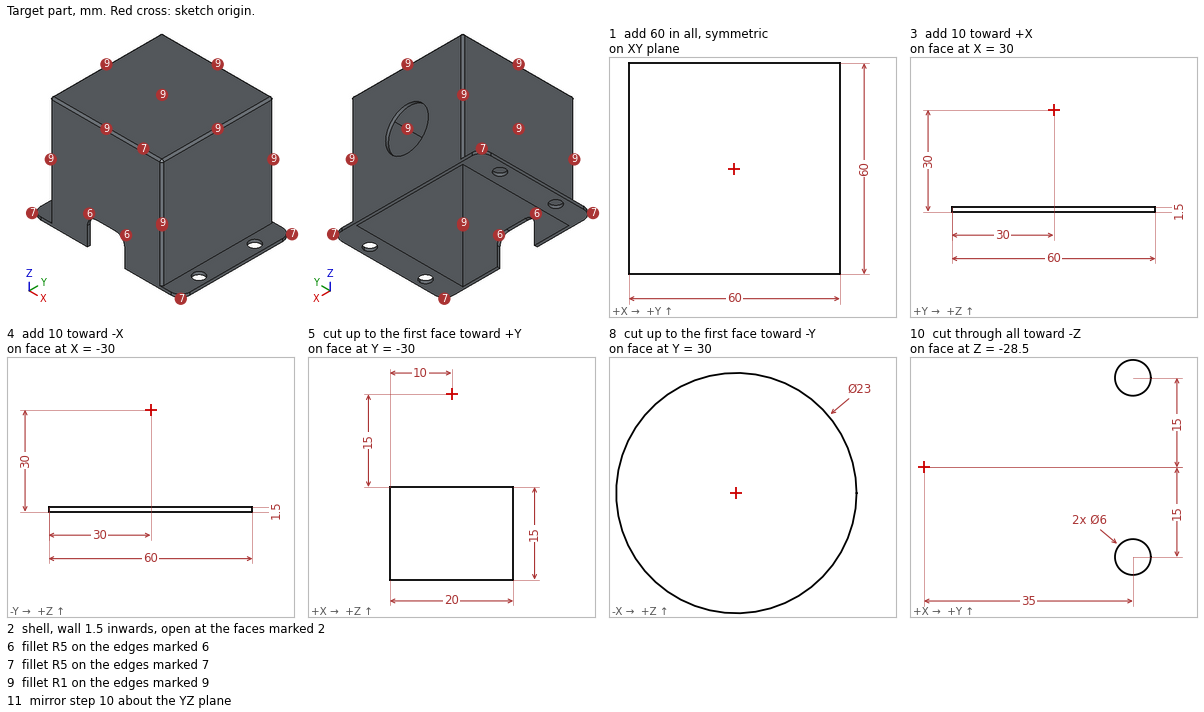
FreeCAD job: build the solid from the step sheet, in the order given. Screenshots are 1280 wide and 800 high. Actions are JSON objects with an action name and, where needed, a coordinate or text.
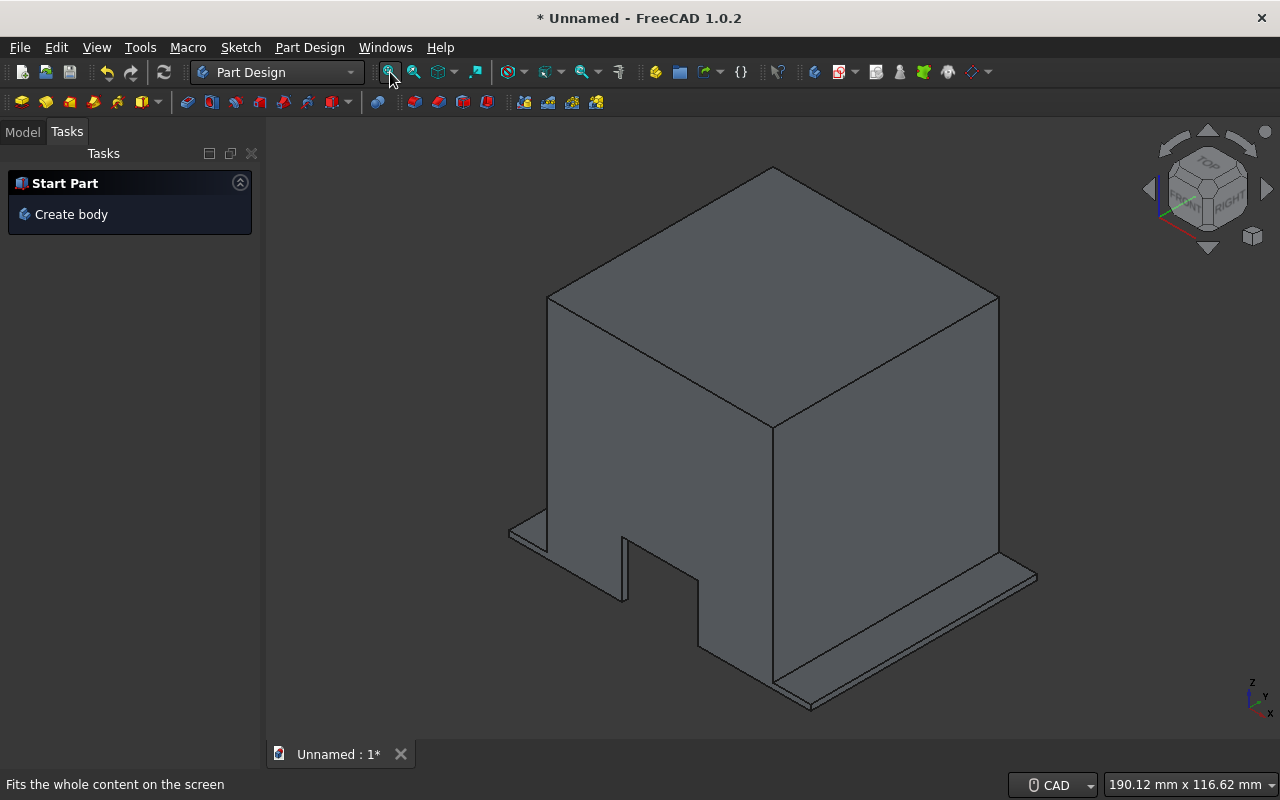
{"action": "key", "text": "2"}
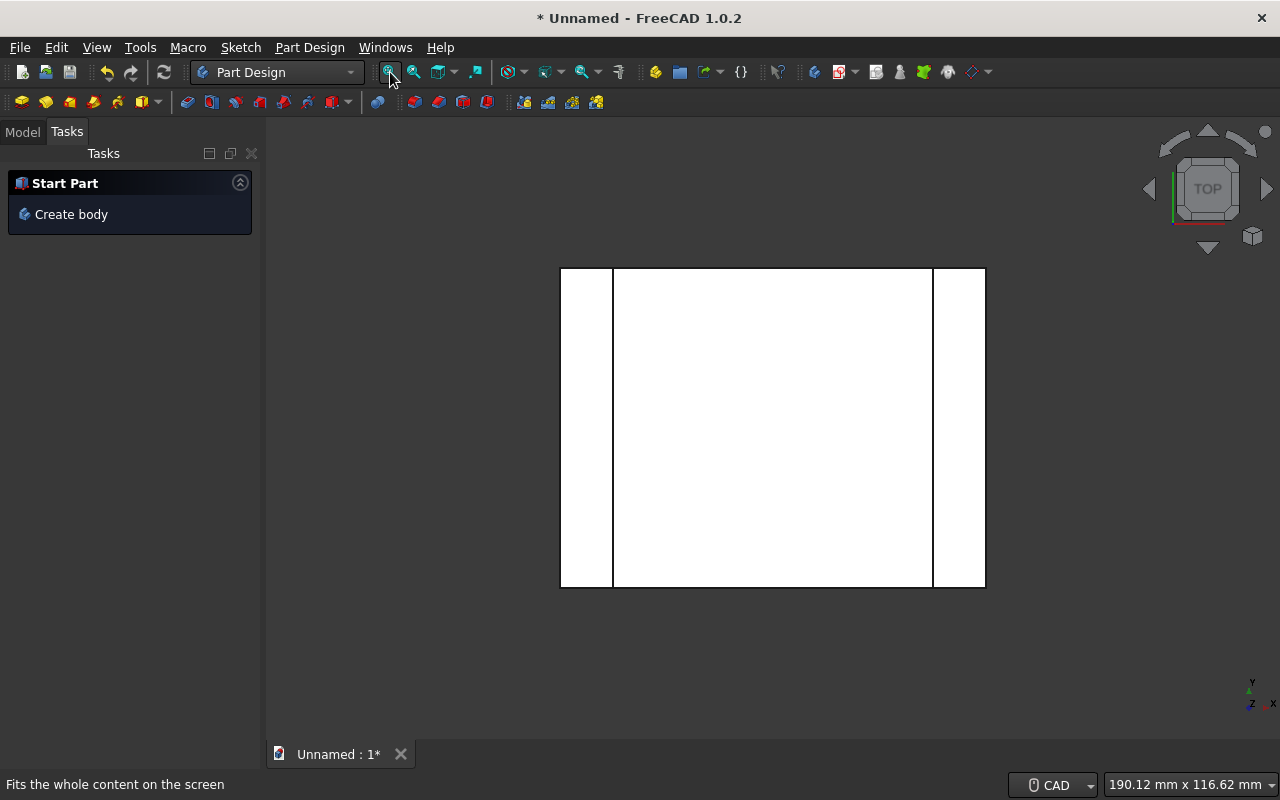
{"action": "scroll", "coordinate": [826, 583], "scroll_direction": "up", "scroll_amount": 9}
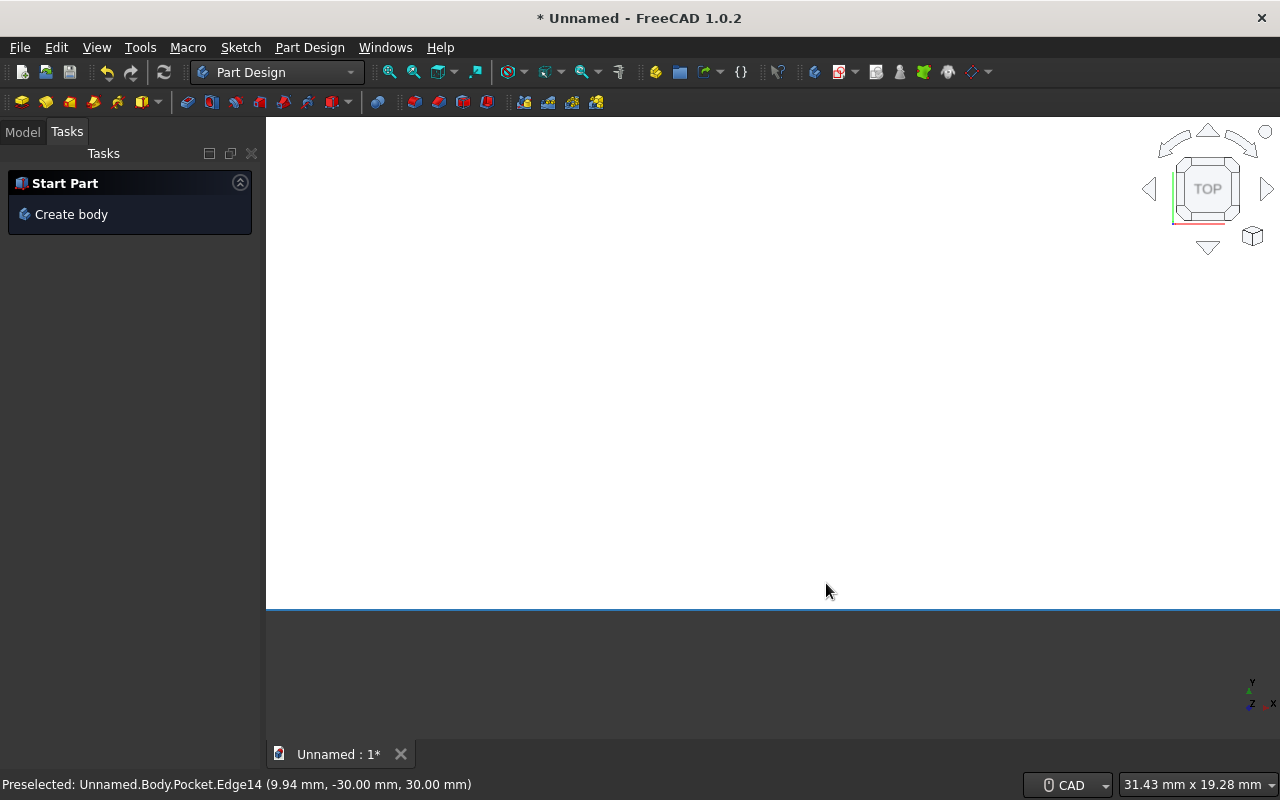
{"action": "key", "text": "v f"}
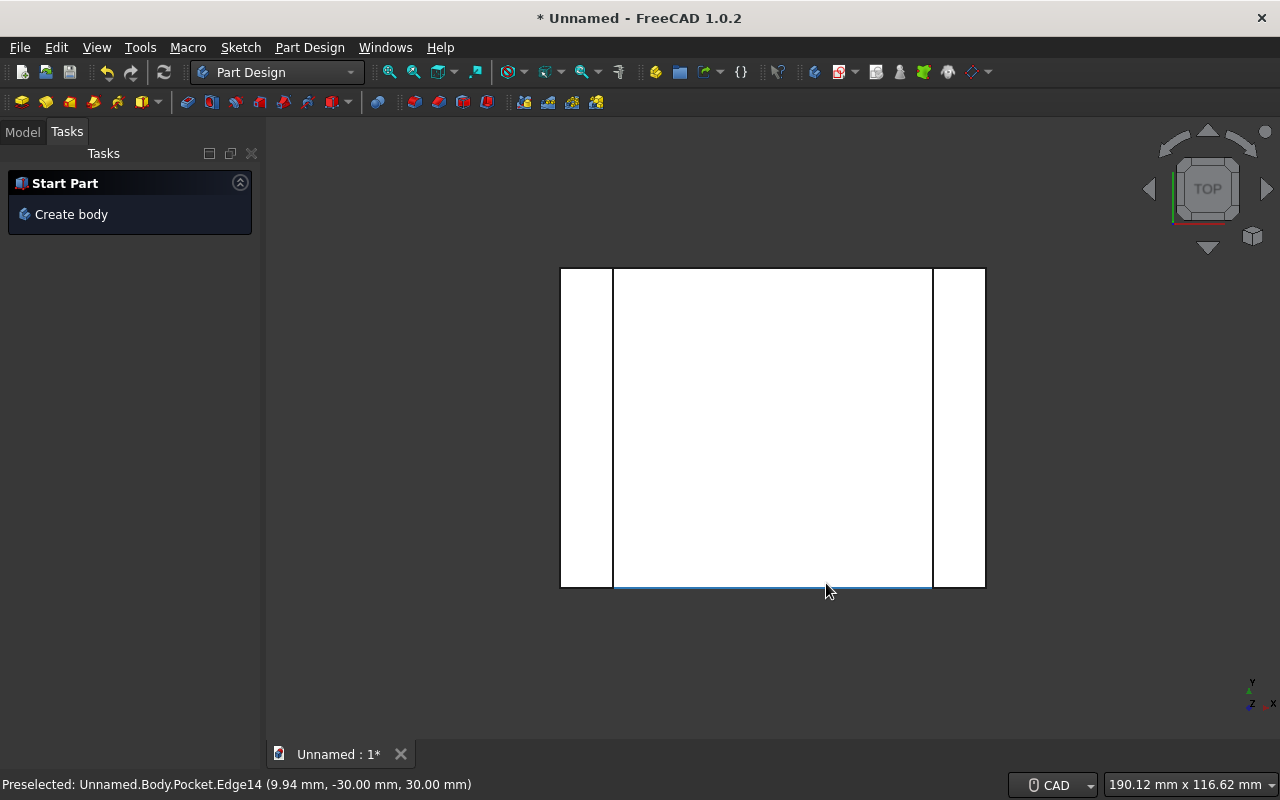
{"action": "key", "text": "0"}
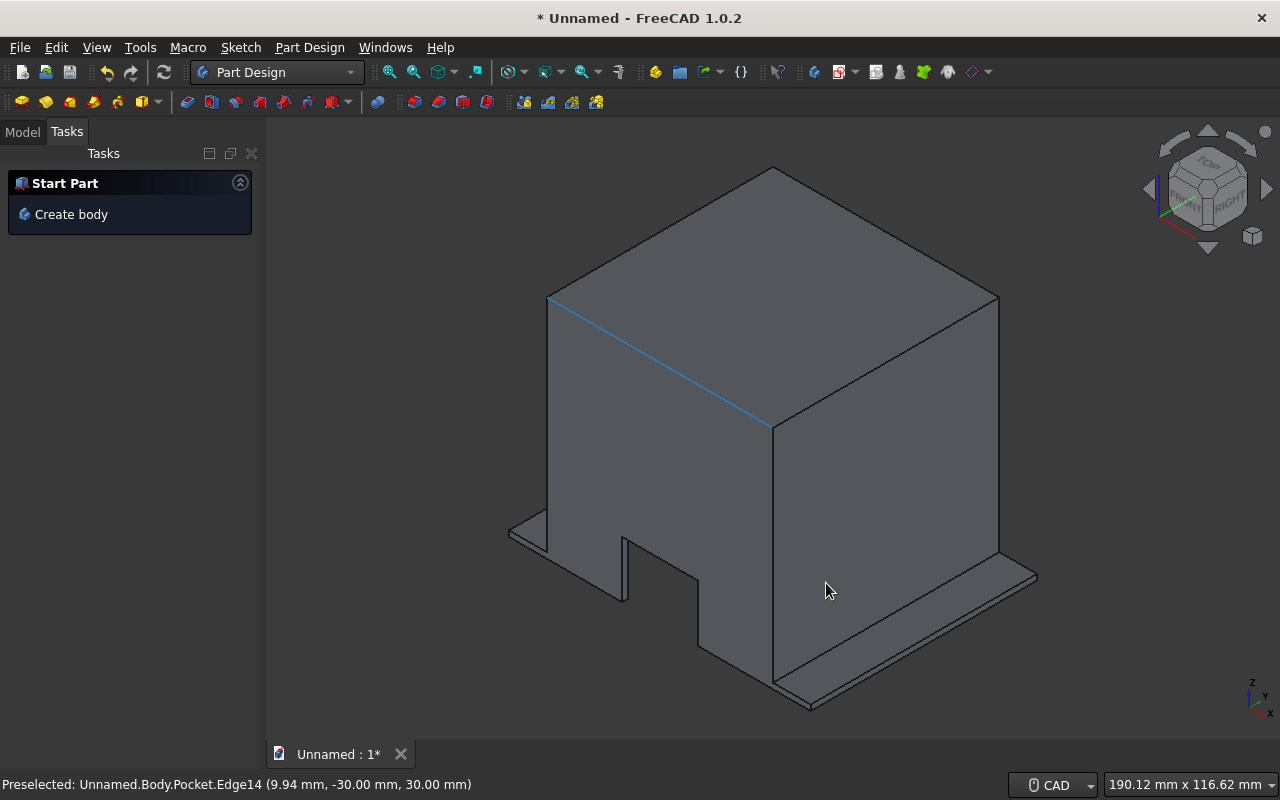
{"action": "scroll", "coordinate": [700, 578], "scroll_direction": "up", "scroll_amount": 9}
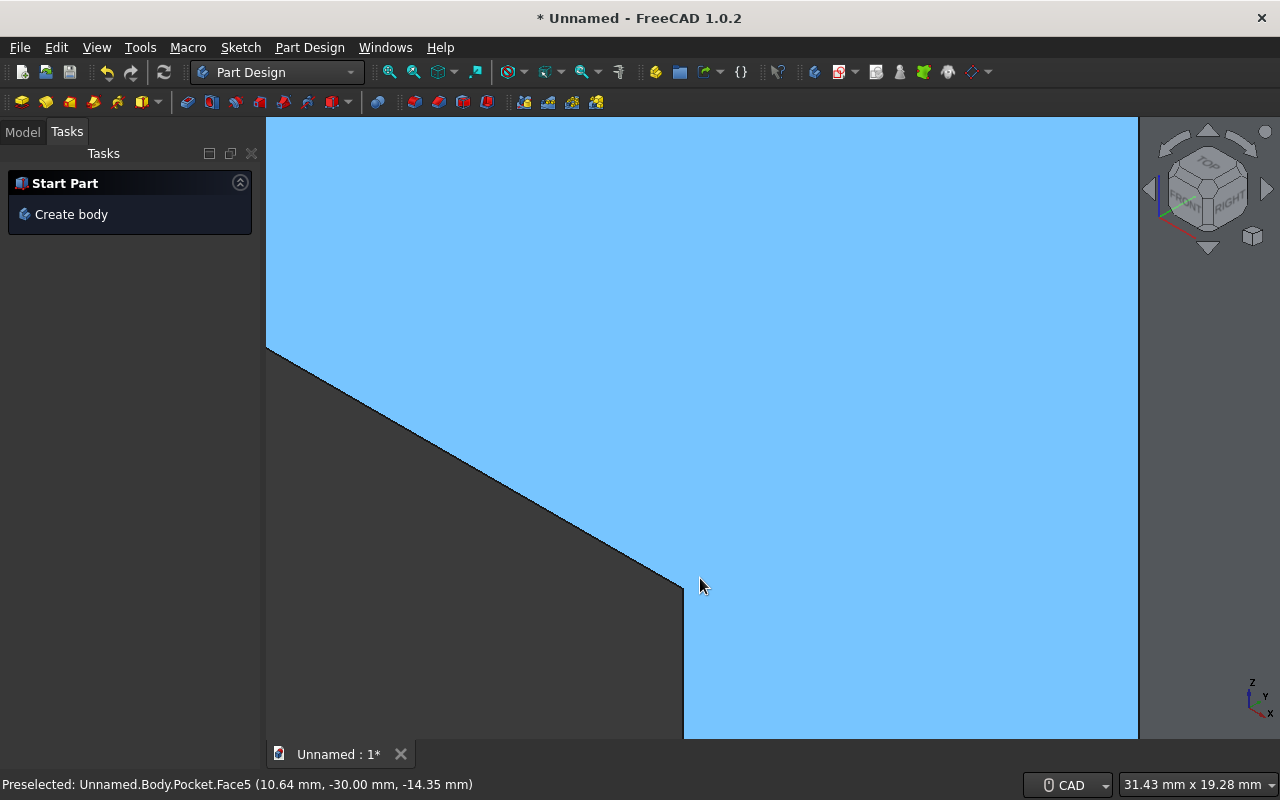
{"action": "left_click", "coordinate": [390, 72]}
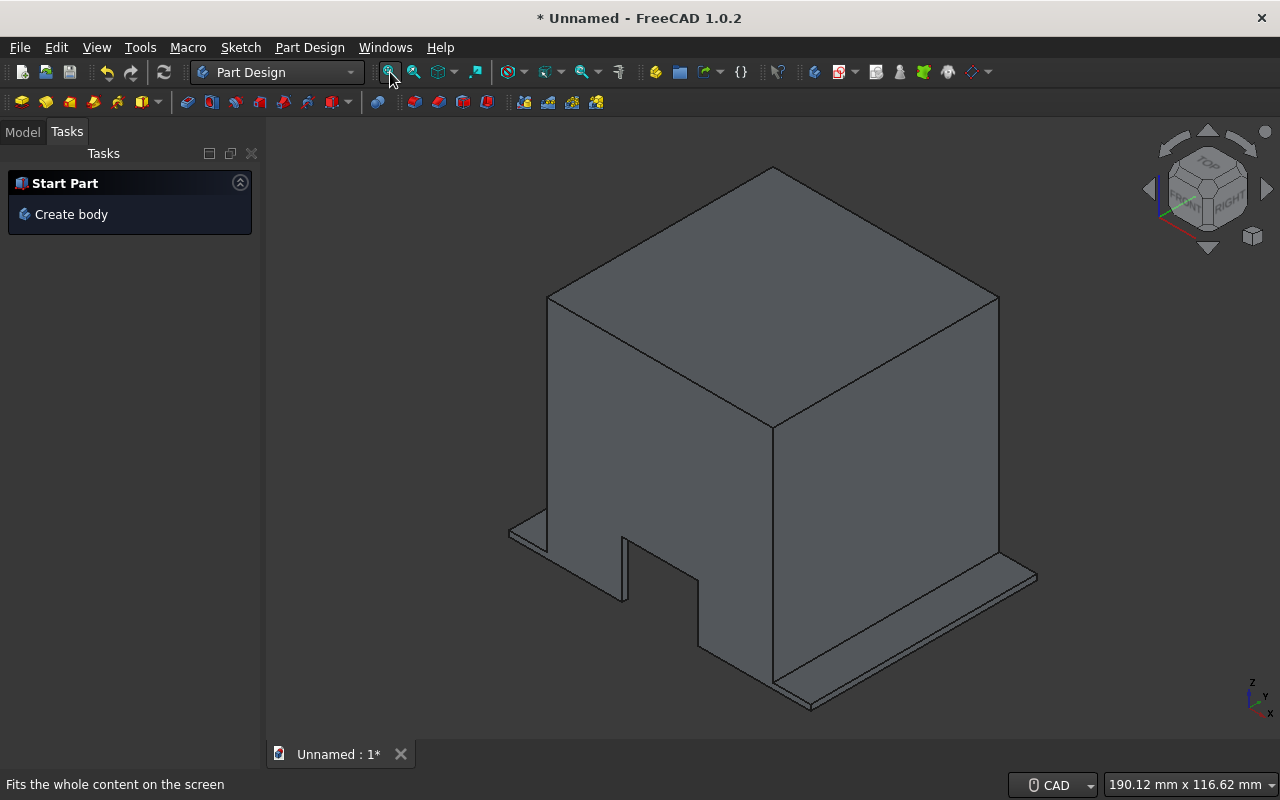
{"action": "key", "text": "1"}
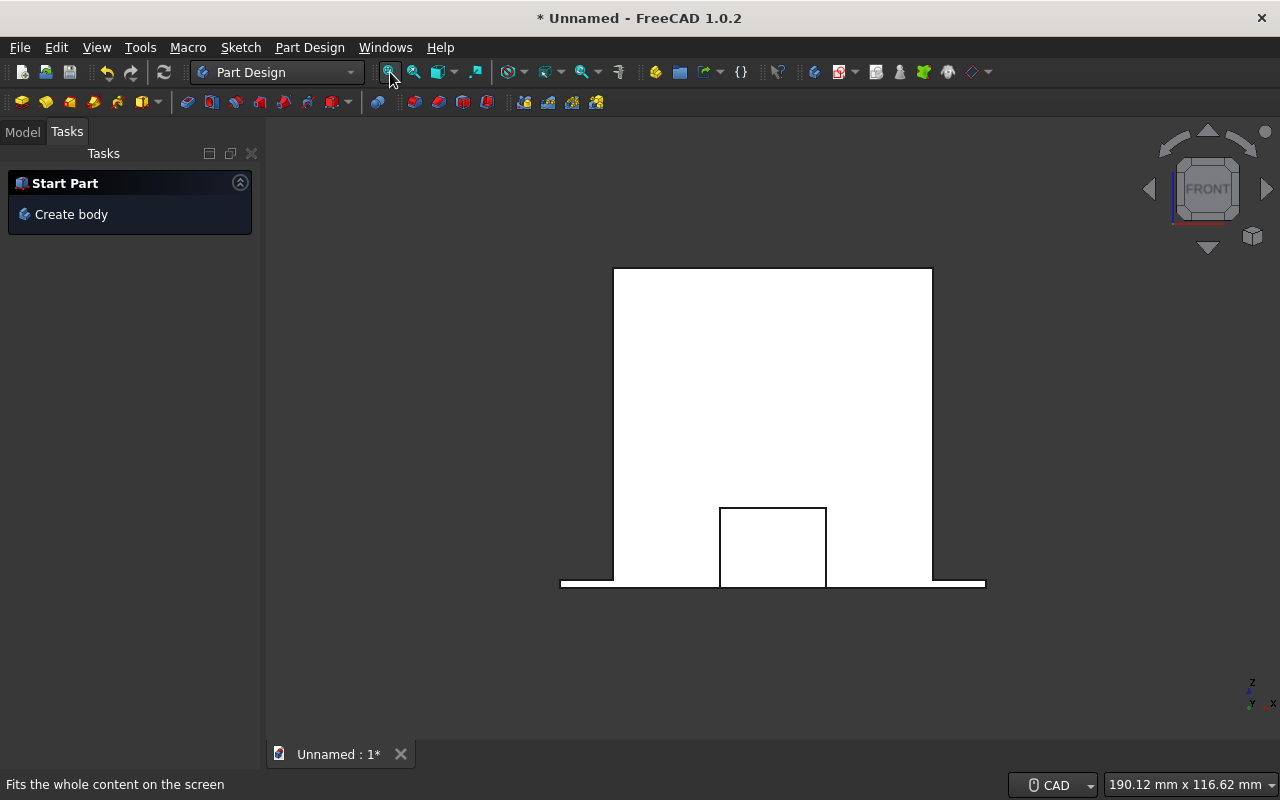
{"action": "scroll", "coordinate": [826, 507], "scroll_direction": "up", "scroll_amount": 9}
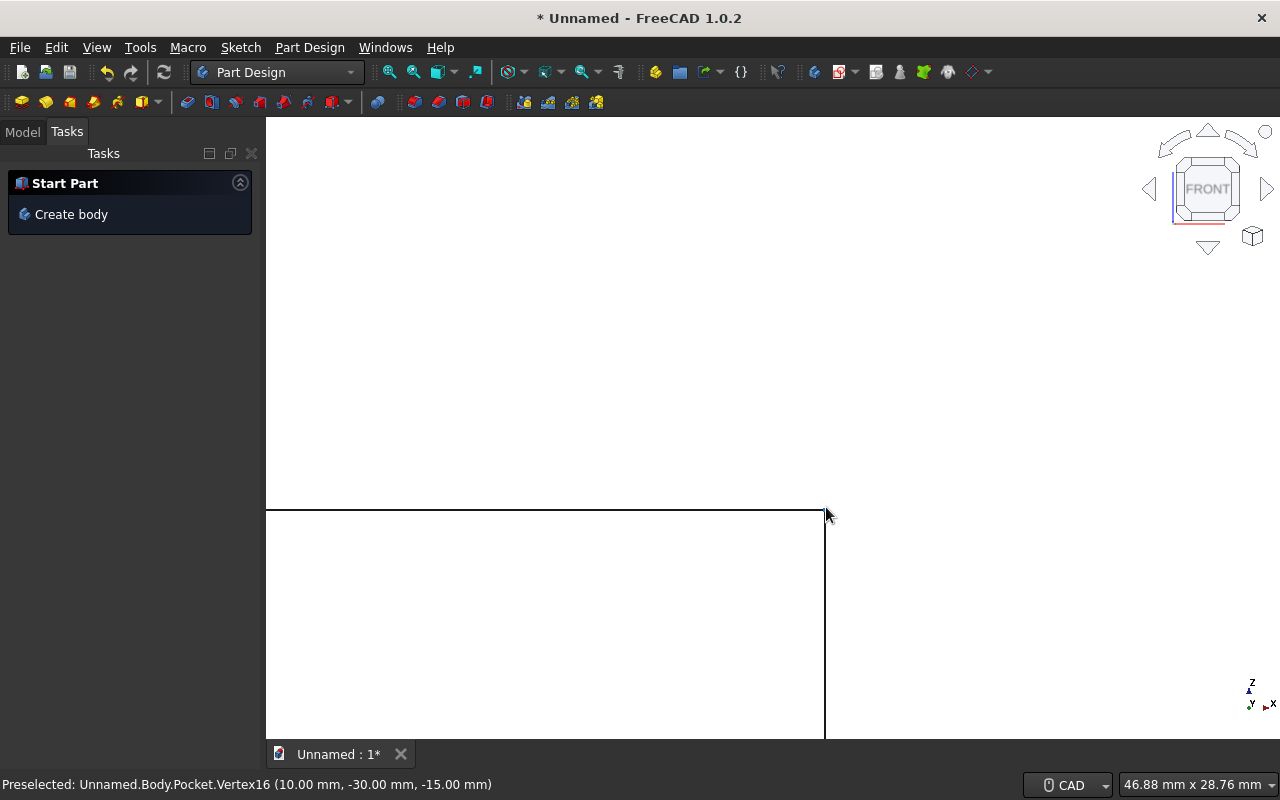
{"action": "key", "text": "v f"}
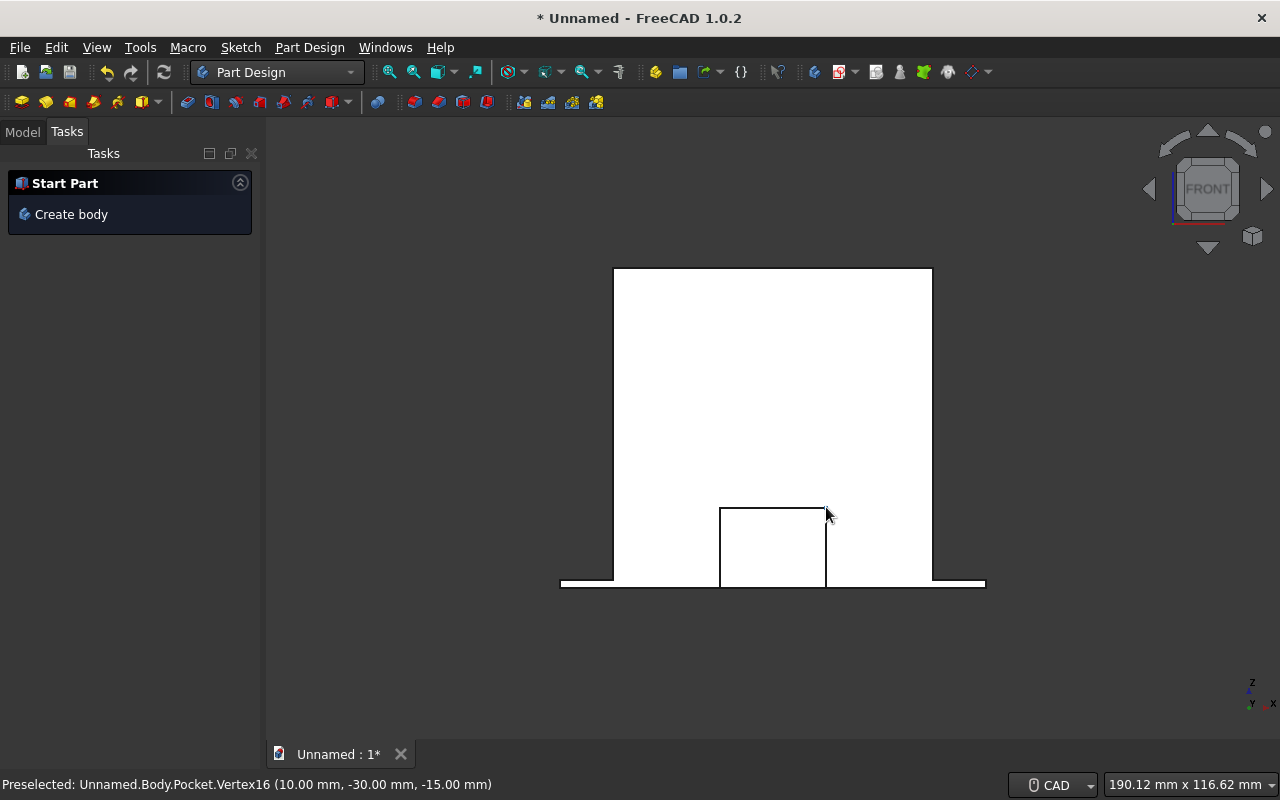
{"action": "key", "text": "3"}